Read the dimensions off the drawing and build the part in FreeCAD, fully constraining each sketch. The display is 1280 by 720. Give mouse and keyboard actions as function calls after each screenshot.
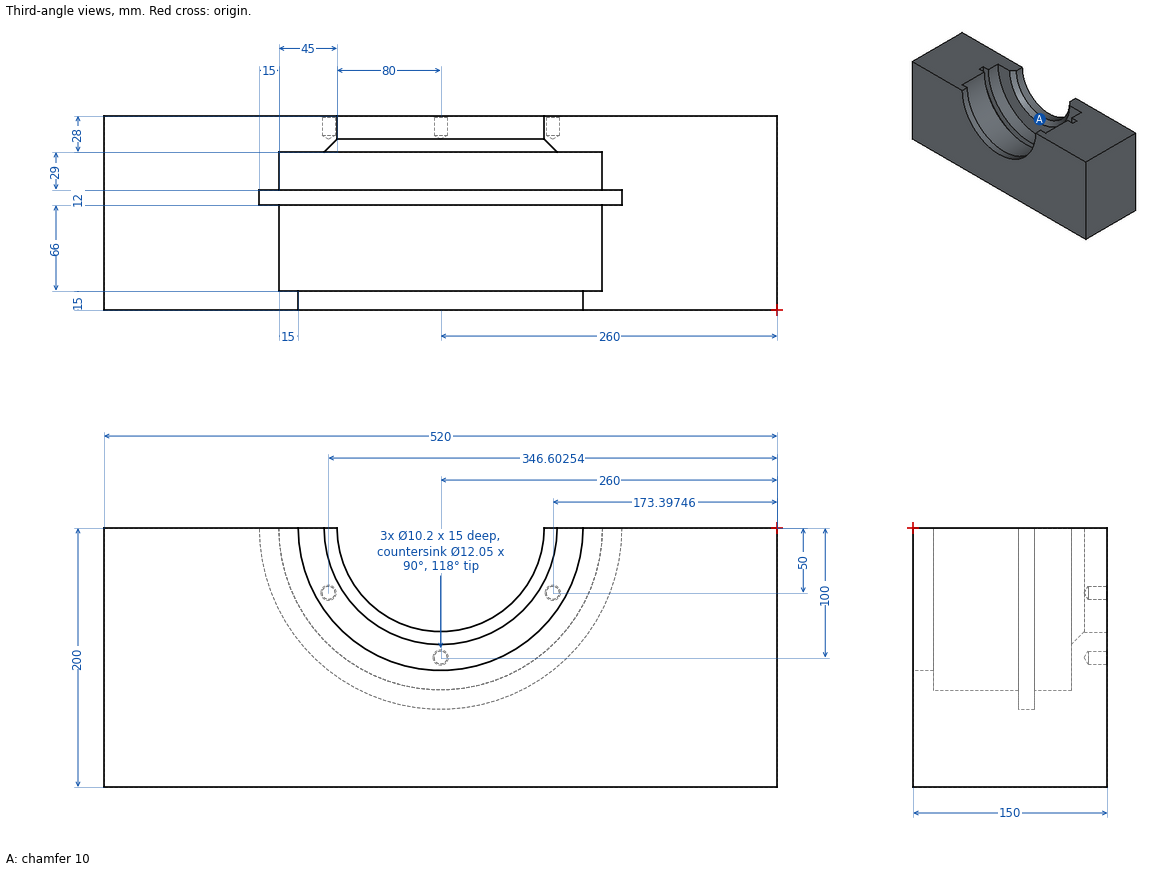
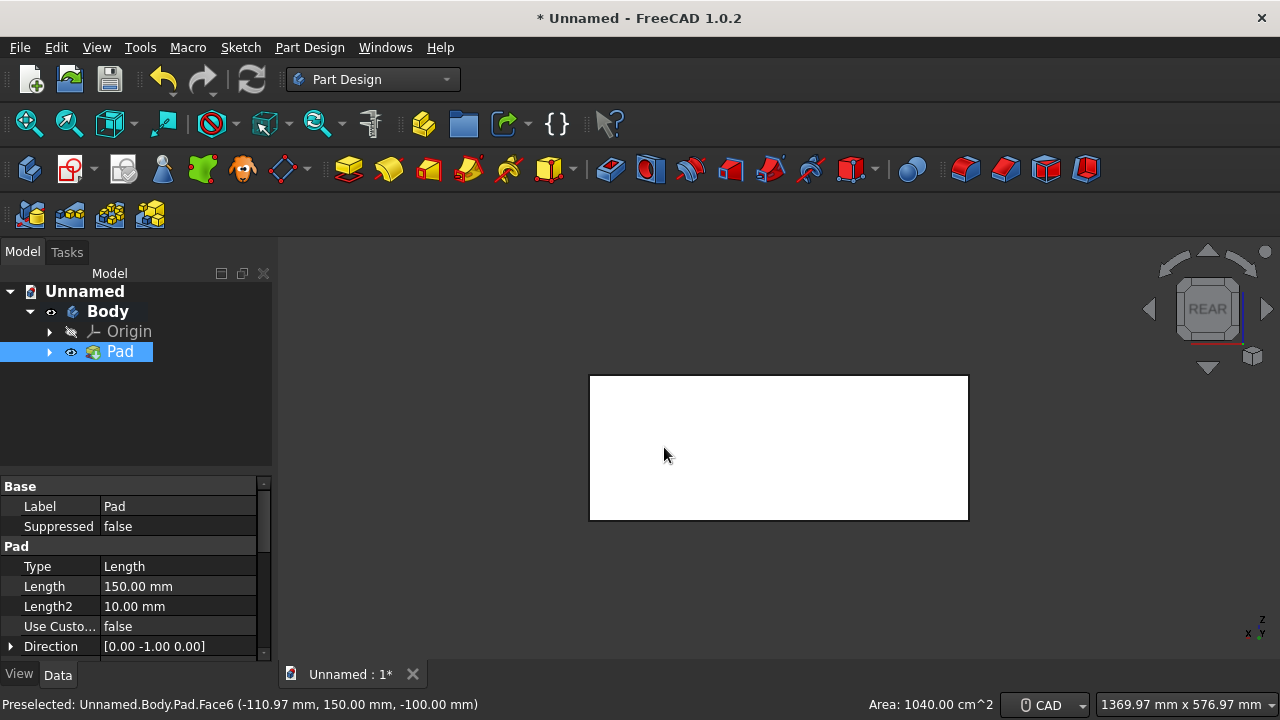
click(70, 170)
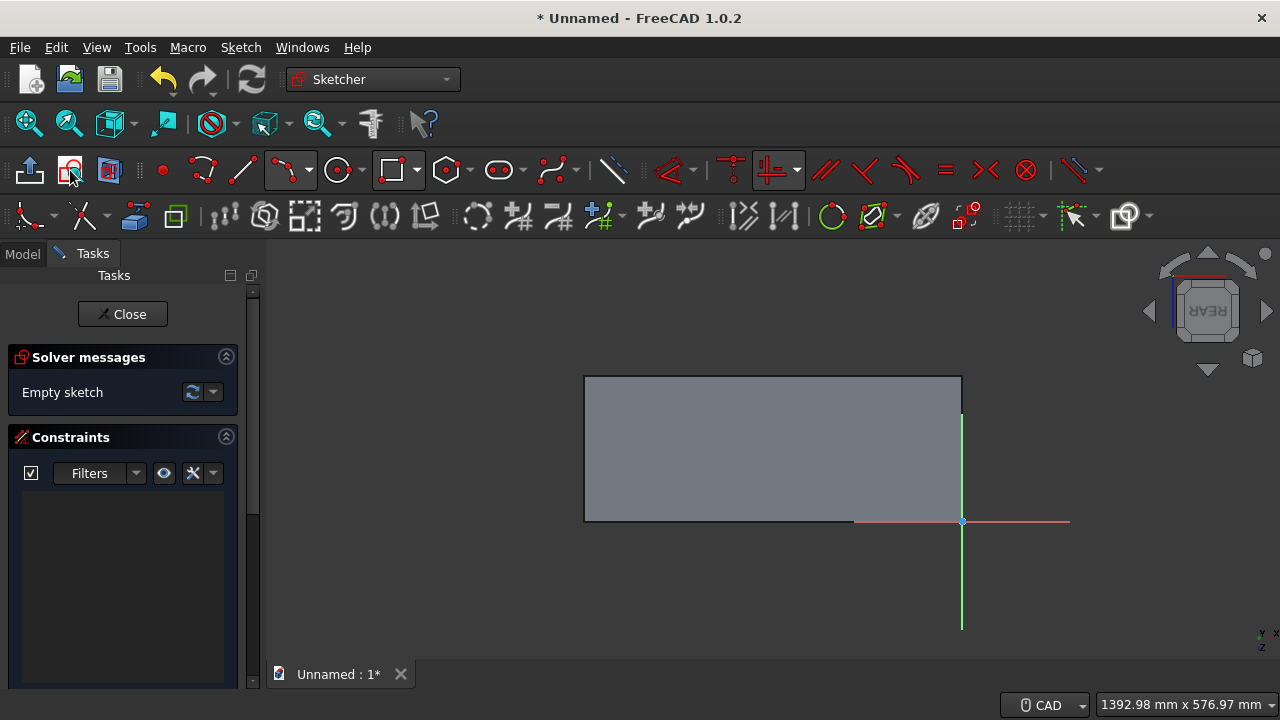
scroll(940, 512, up, 4)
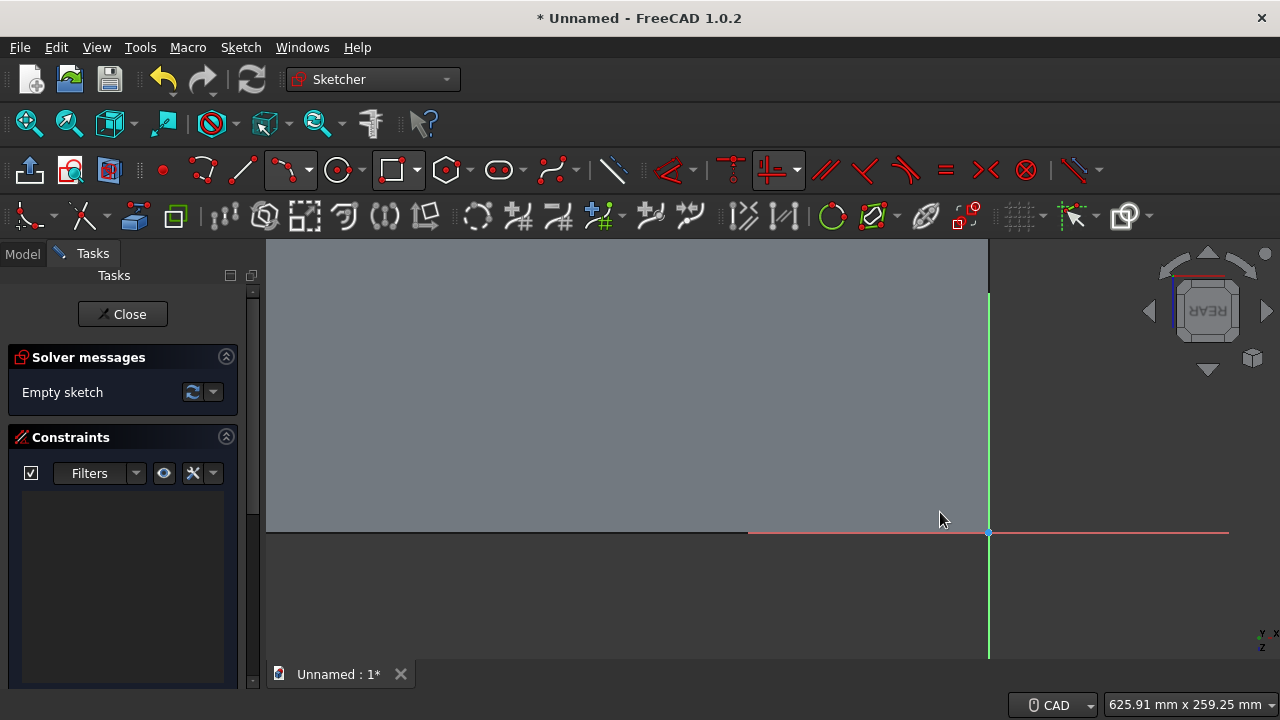
key(g)
key(c)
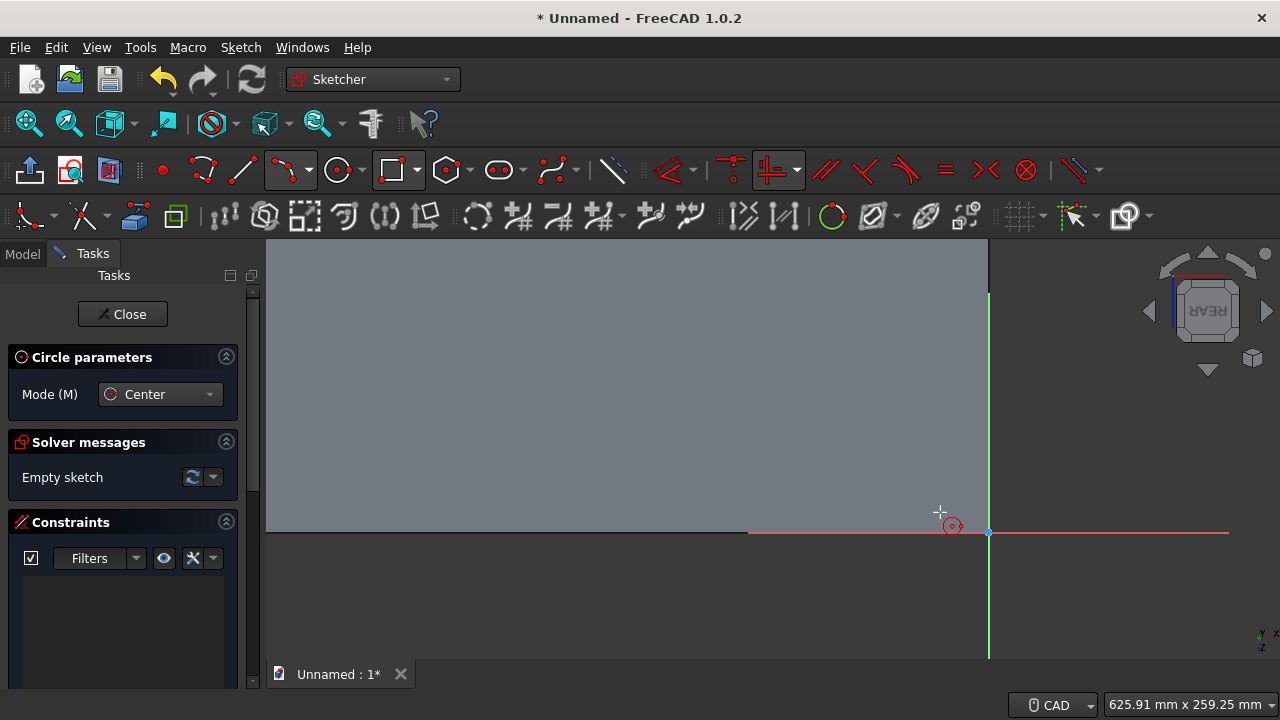
scroll(568, 371, up, 6)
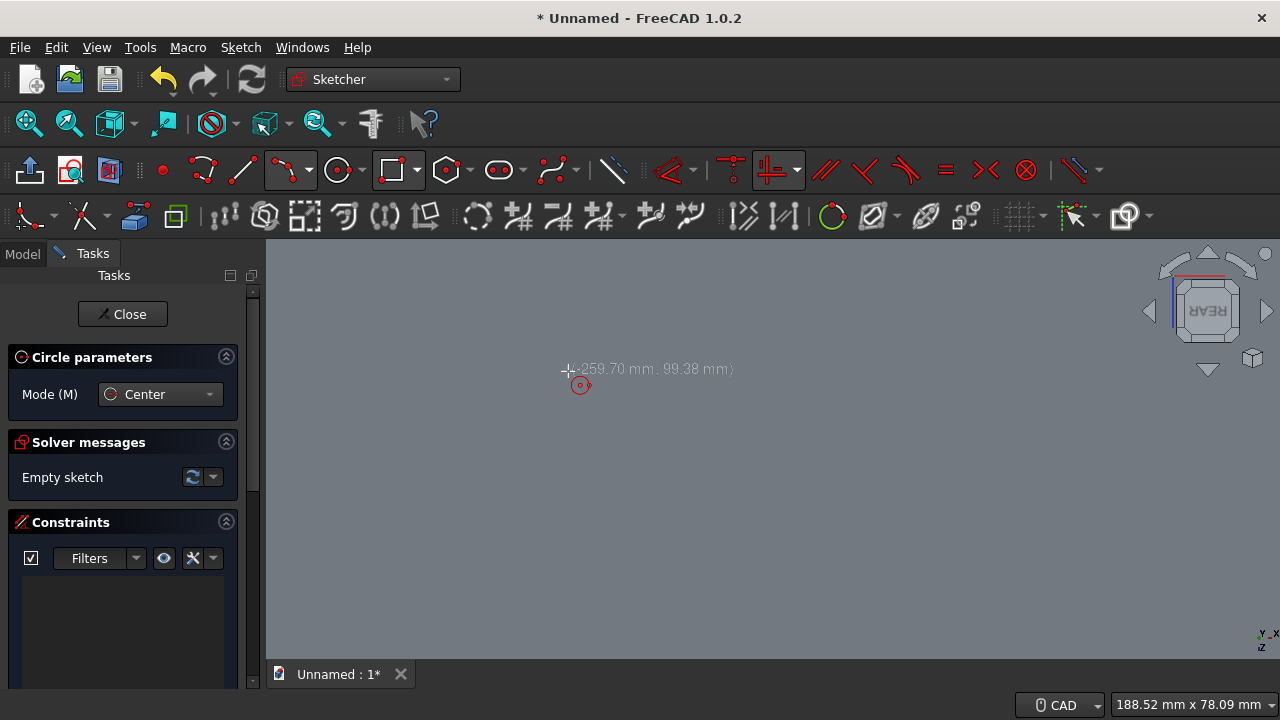
click(566, 370)
click(585, 351)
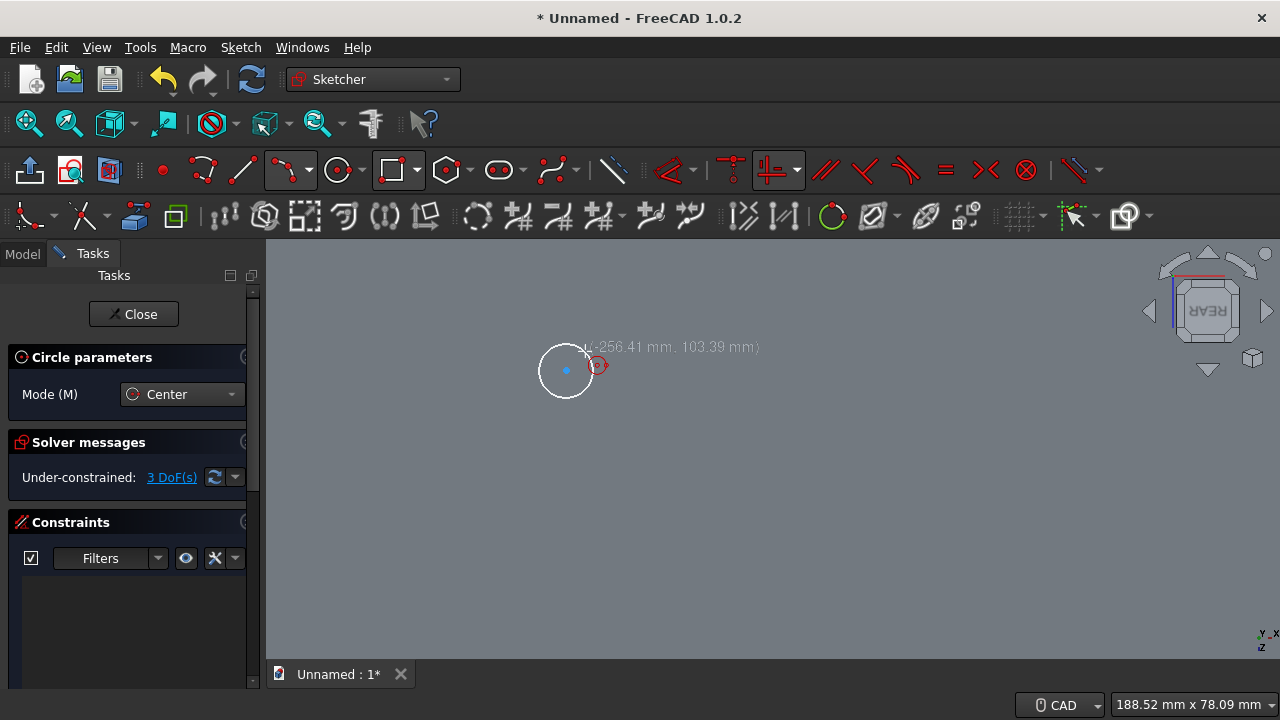
scroll(569, 373, down, 6)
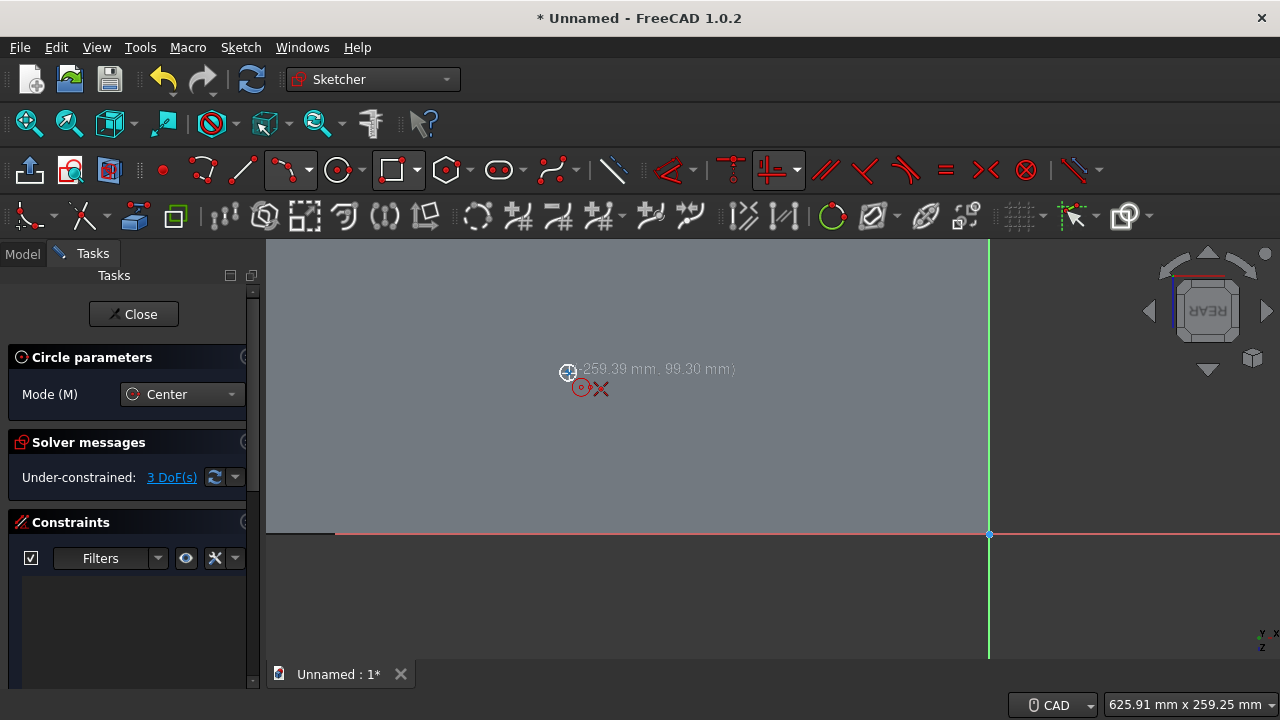
scroll(709, 453, up, 6)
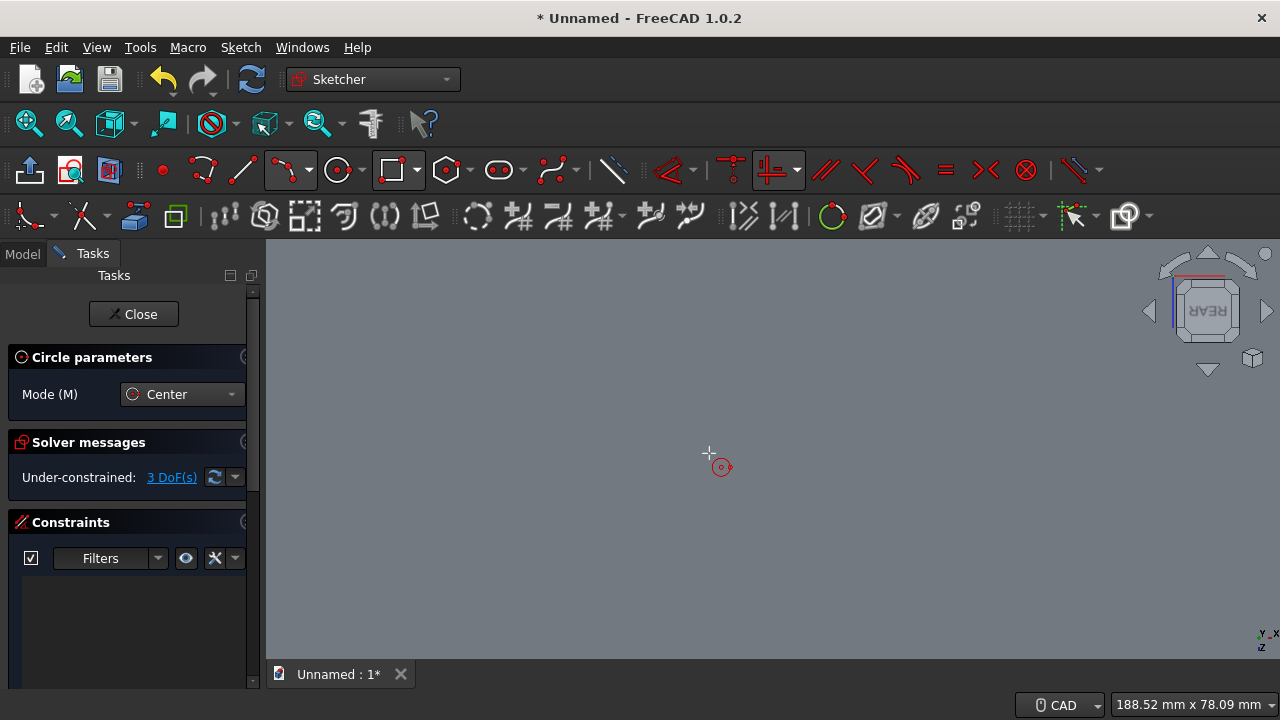
click(706, 453)
click(726, 434)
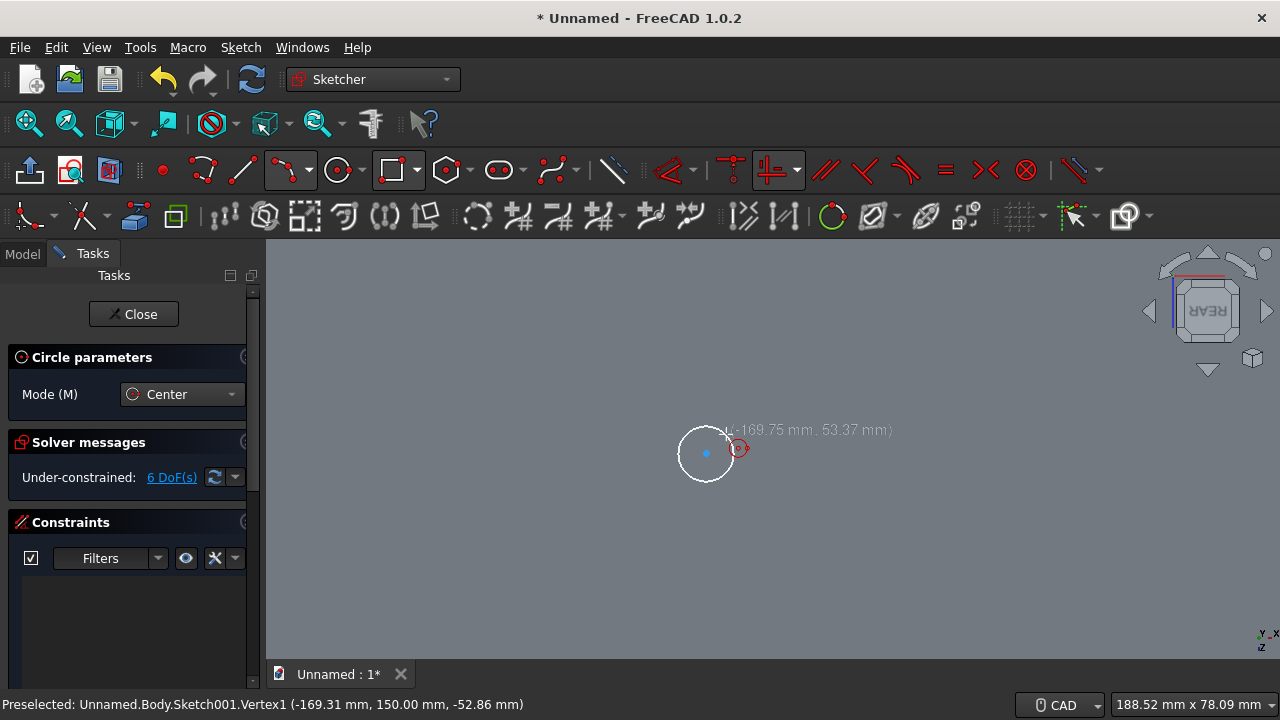
scroll(709, 453, down, 6)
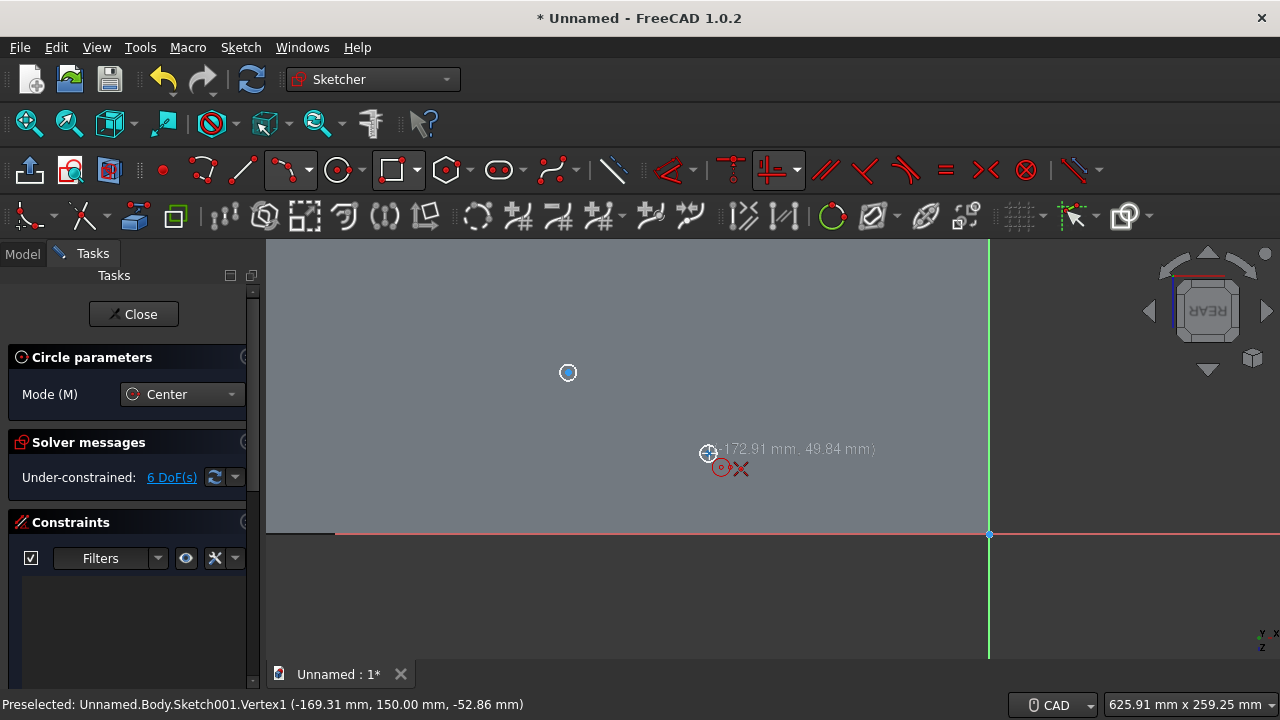
scroll(428, 453, up, 6)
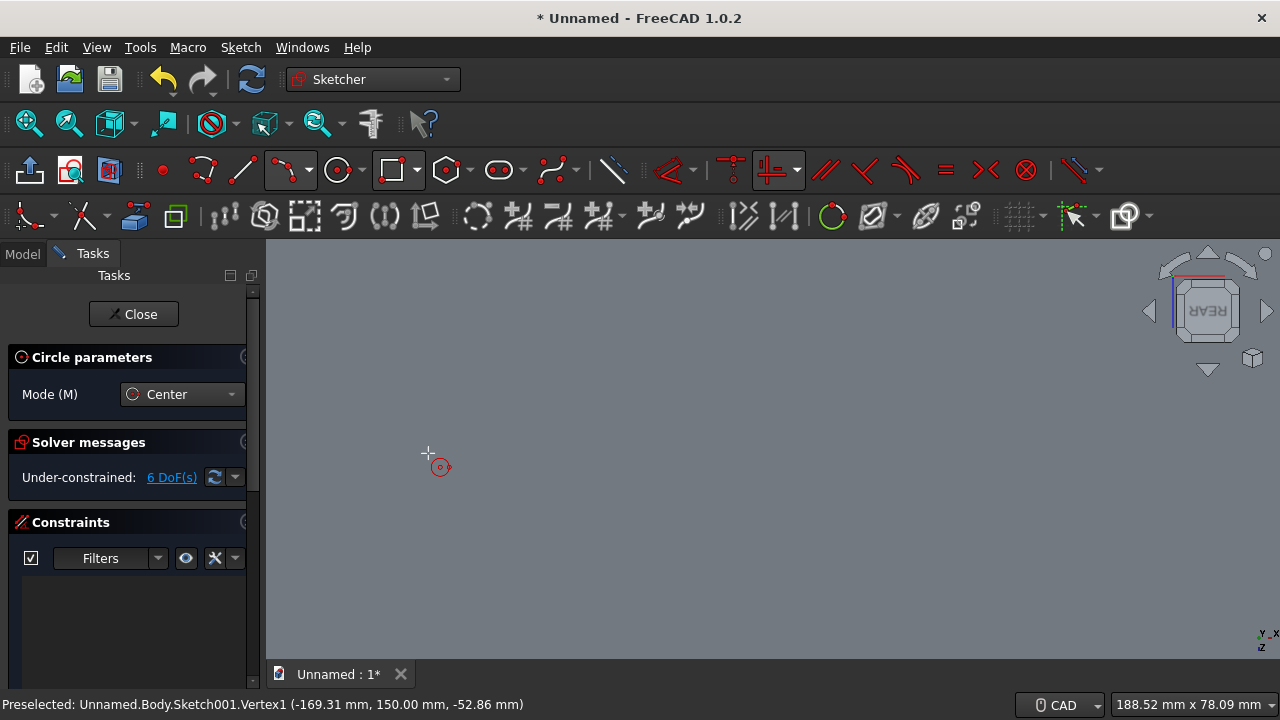
click(427, 453)
click(447, 434)
key(Escape)